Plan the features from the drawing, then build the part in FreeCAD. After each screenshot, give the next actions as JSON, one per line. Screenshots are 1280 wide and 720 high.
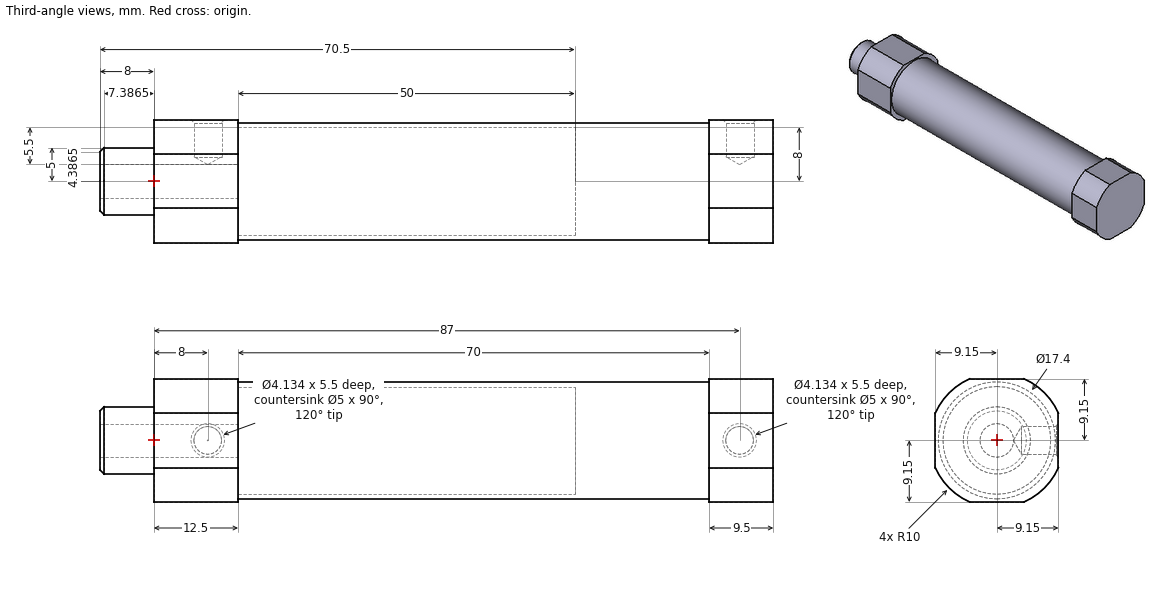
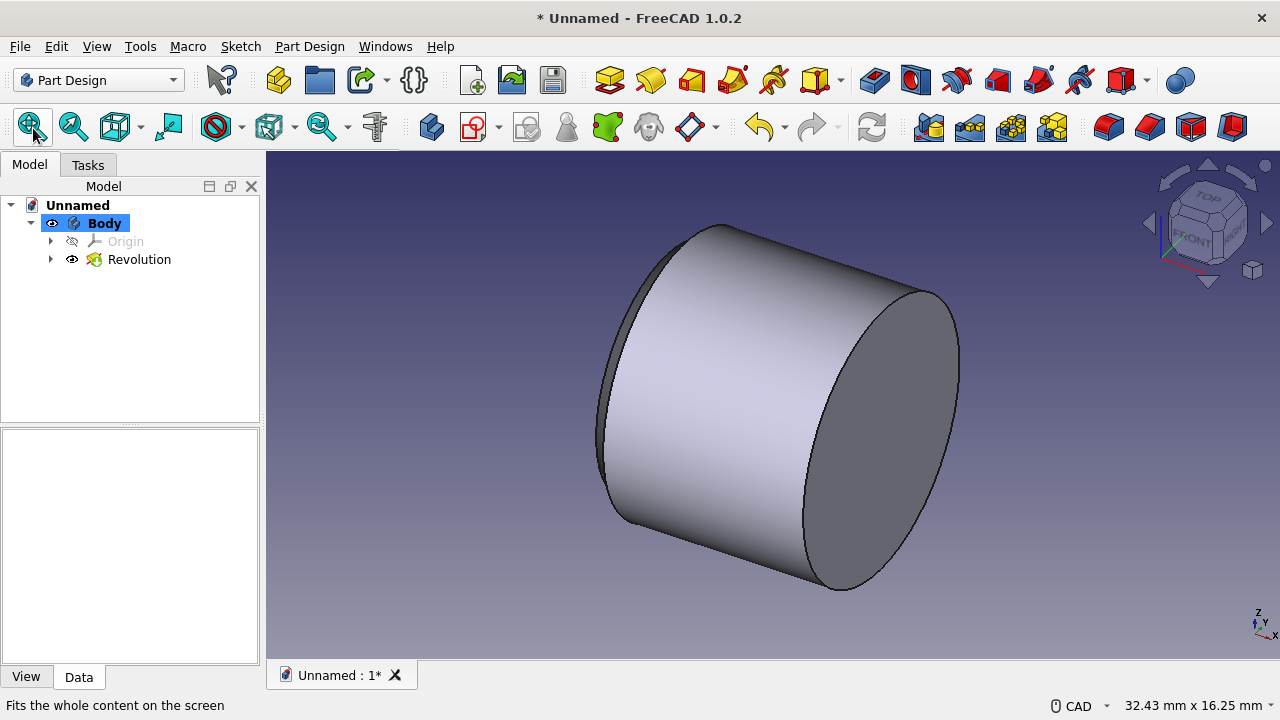
{"action": "left_click", "coordinate": [881, 440]}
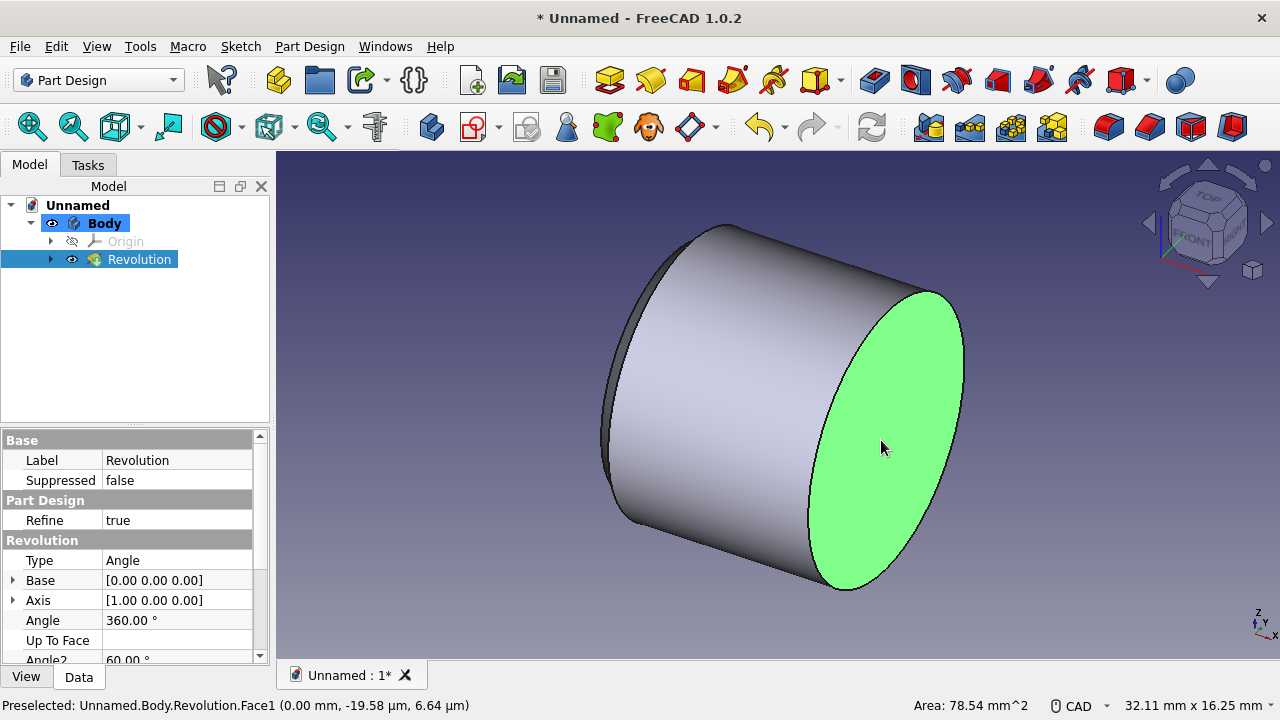
{"action": "left_click", "coordinate": [472, 128]}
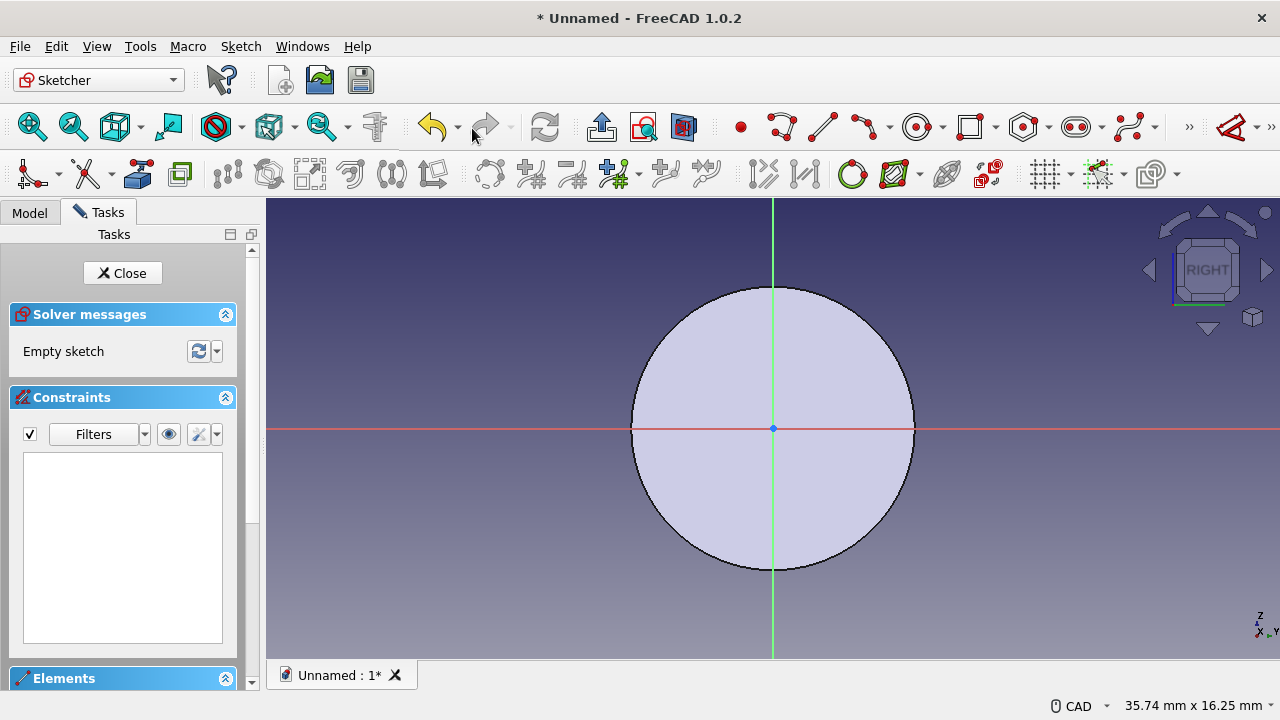
{"action": "scroll", "coordinate": [621, 428], "scroll_direction": "down", "scroll_amount": 3}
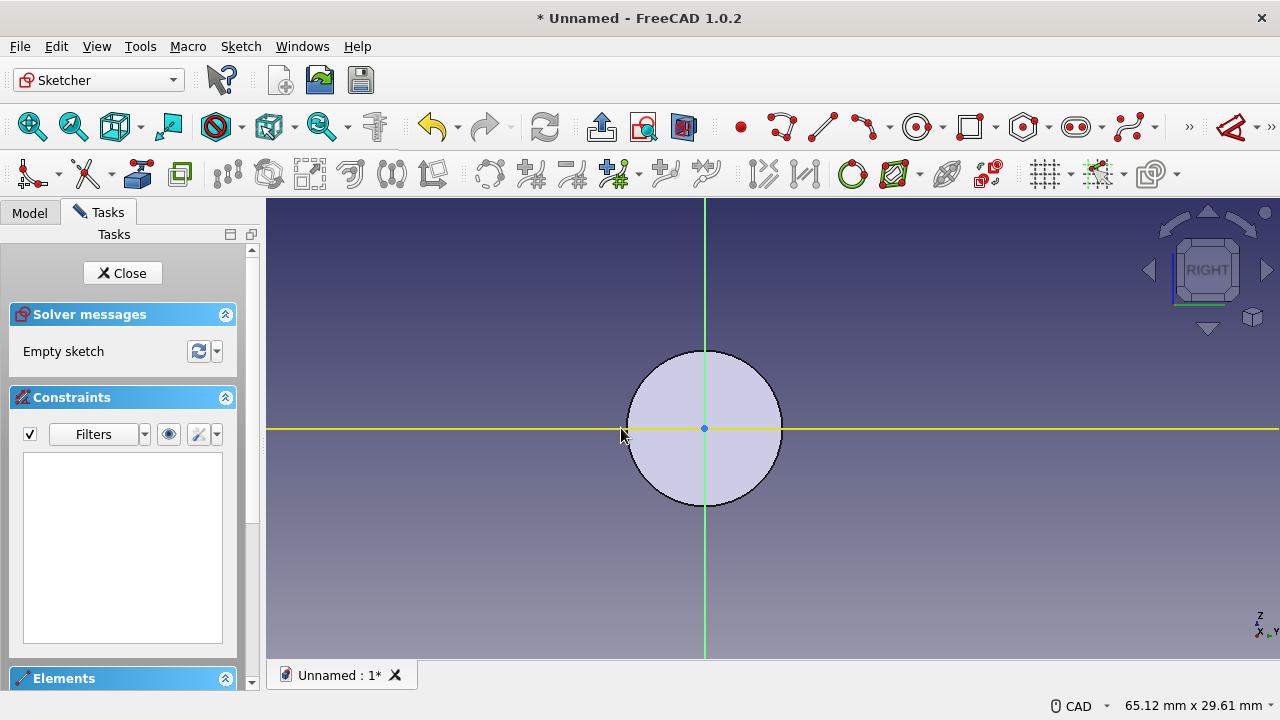
{"action": "key", "text": "g l"}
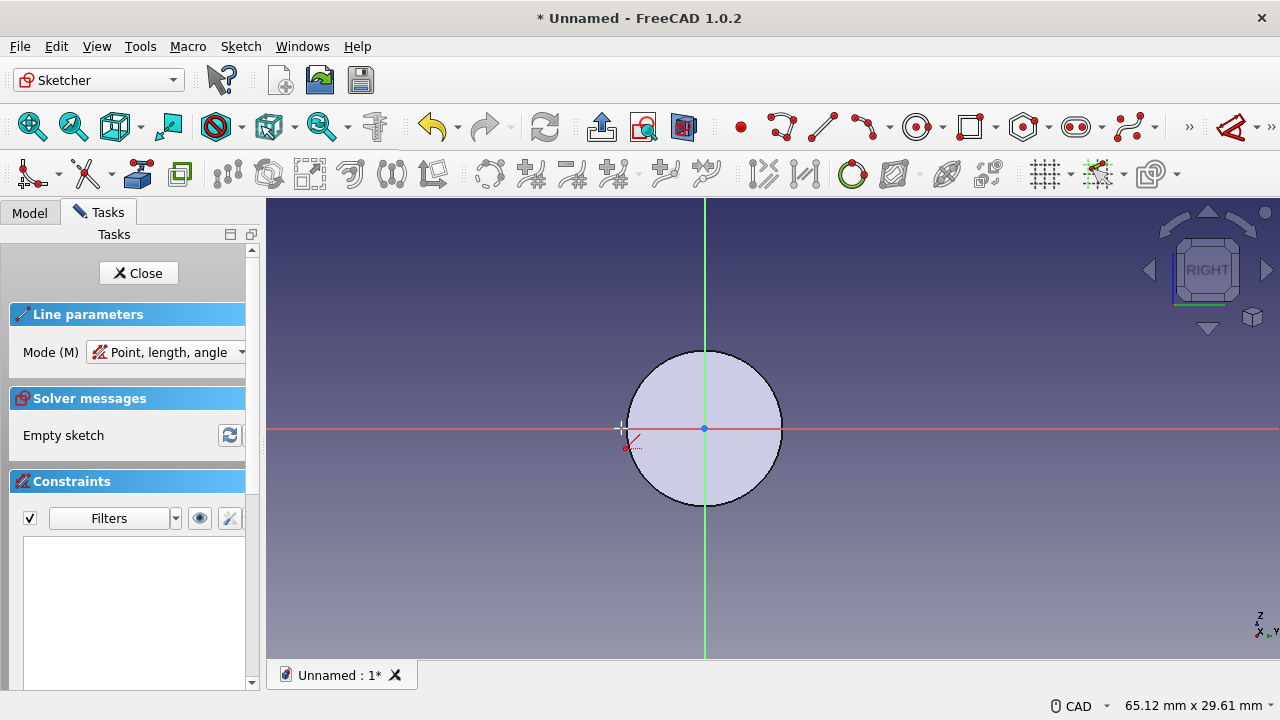
{"action": "left_click", "coordinate": [562, 366]}
{"action": "left_click", "coordinate": [562, 491]}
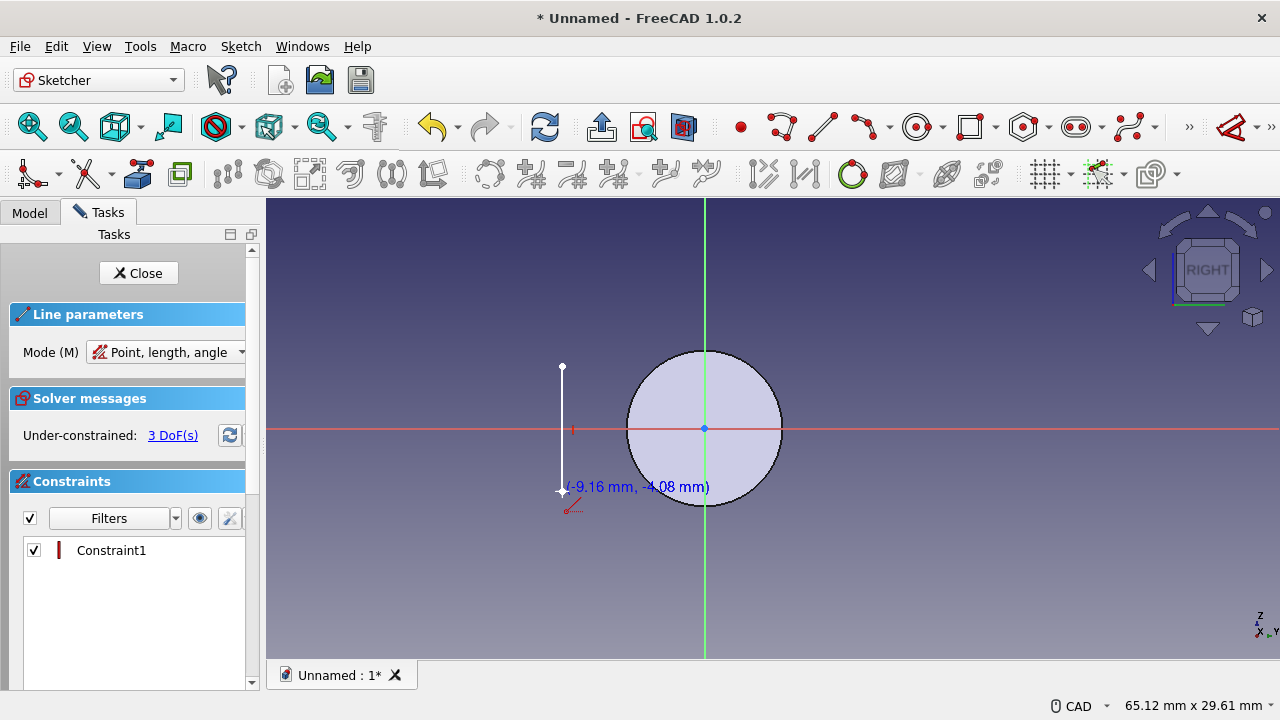
{"action": "left_click", "coordinate": [642, 571]}
{"action": "left_click", "coordinate": [767, 571]}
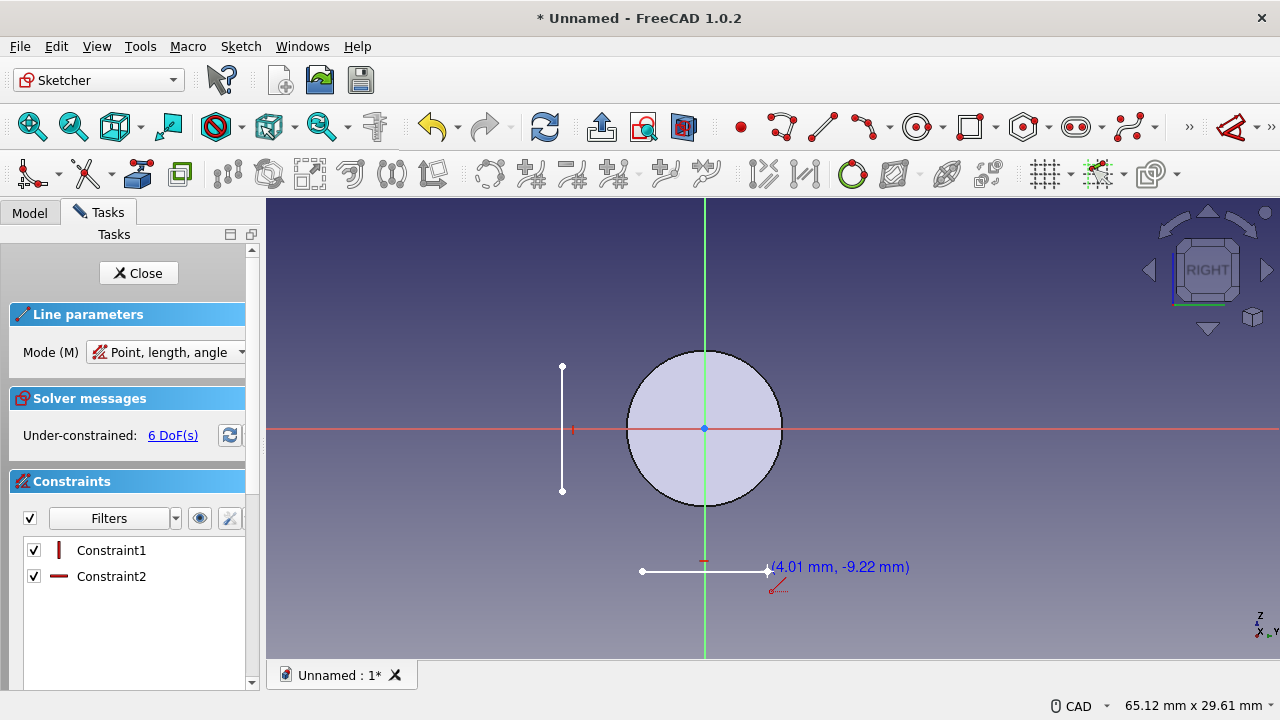
{"action": "left_click", "coordinate": [847, 491]}
{"action": "left_click", "coordinate": [847, 366]}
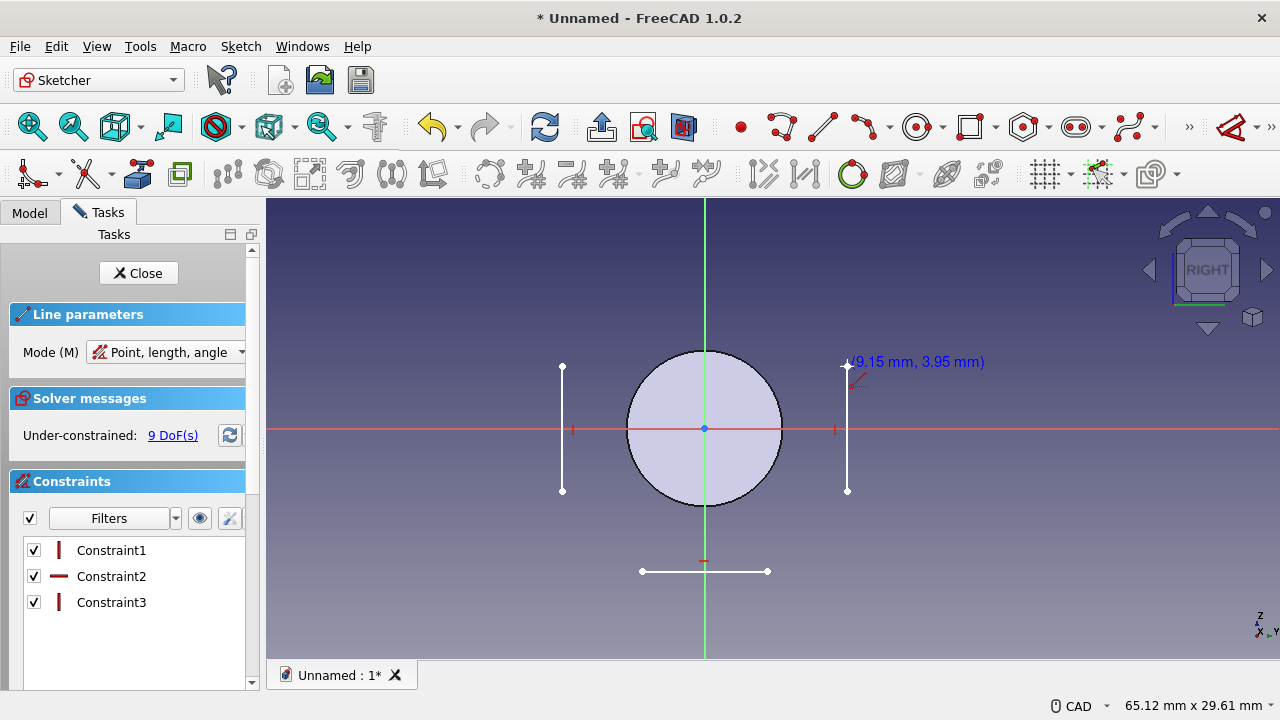
{"action": "left_click", "coordinate": [767, 286]}
{"action": "left_click", "coordinate": [642, 286]}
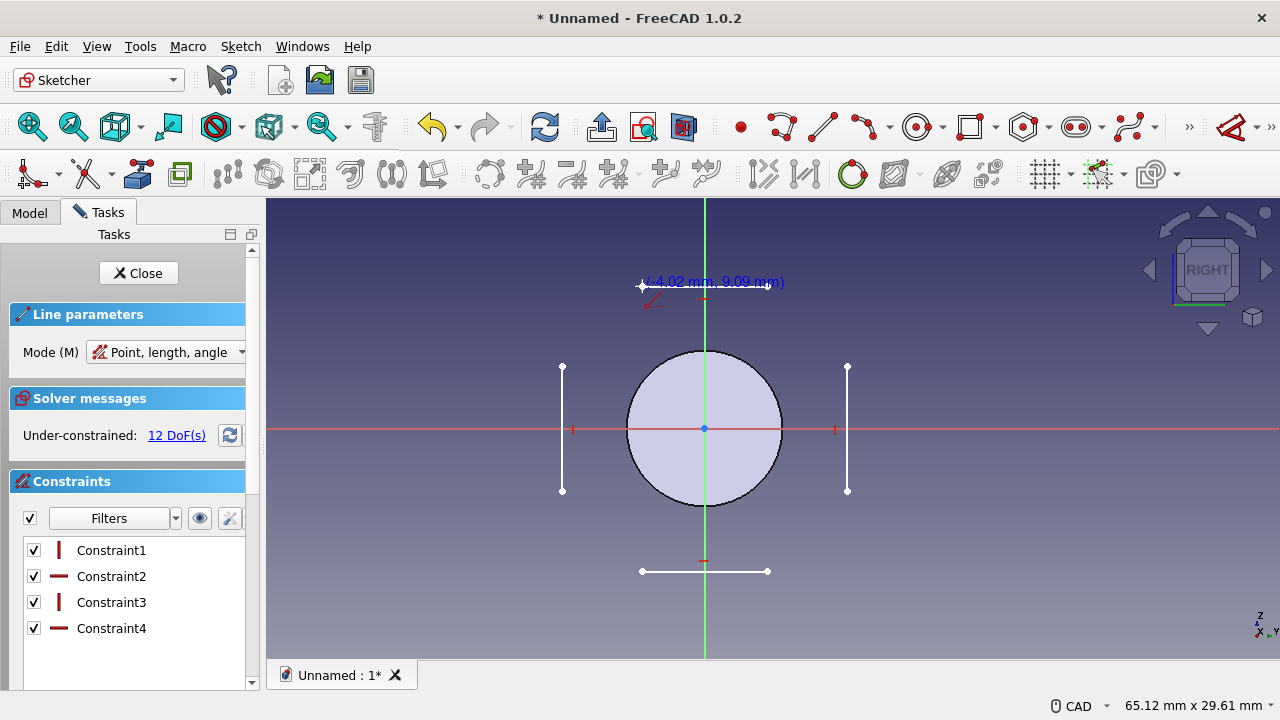
{"action": "left_click", "coordinate": [864, 128]}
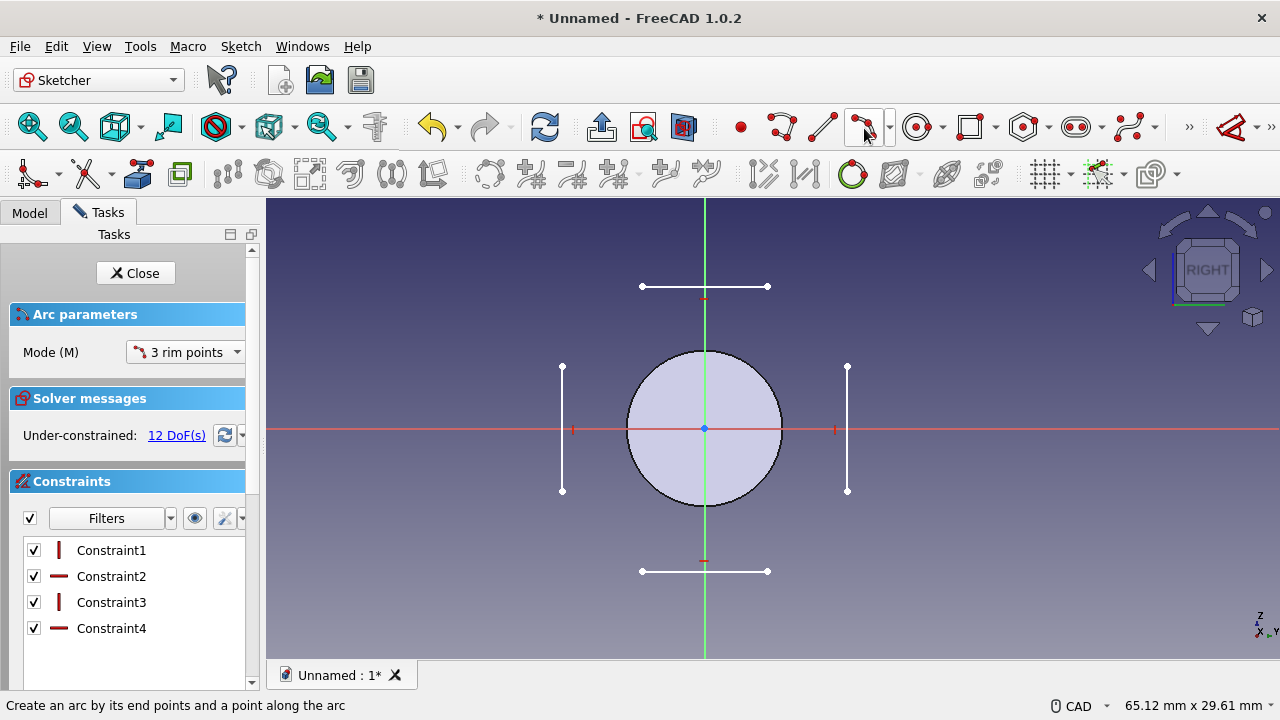
{"action": "left_click", "coordinate": [562, 492]}
{"action": "left_click", "coordinate": [642, 572]}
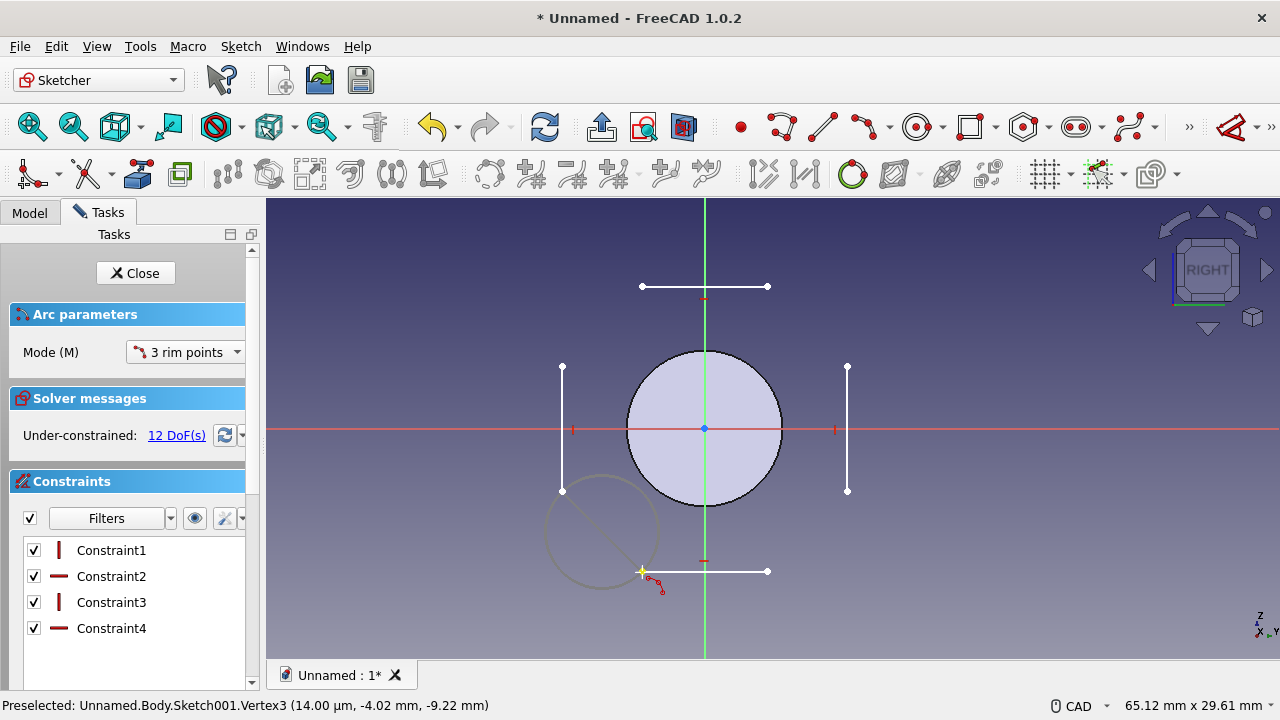
{"action": "scroll", "coordinate": [594, 539], "scroll_direction": "up", "scroll_amount": 3}